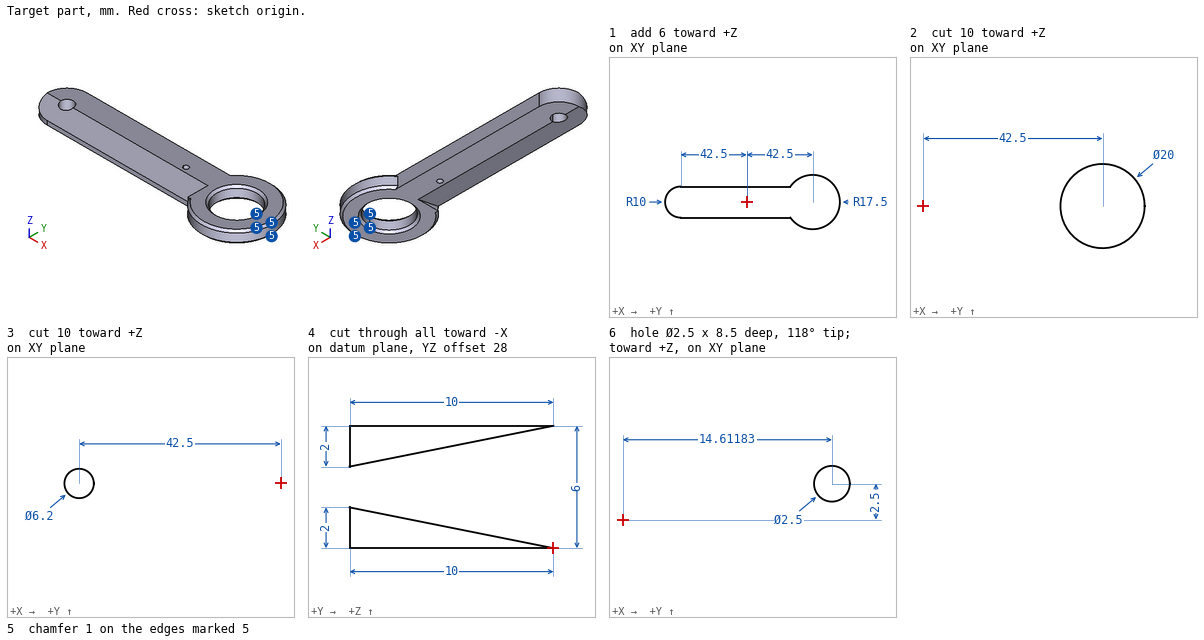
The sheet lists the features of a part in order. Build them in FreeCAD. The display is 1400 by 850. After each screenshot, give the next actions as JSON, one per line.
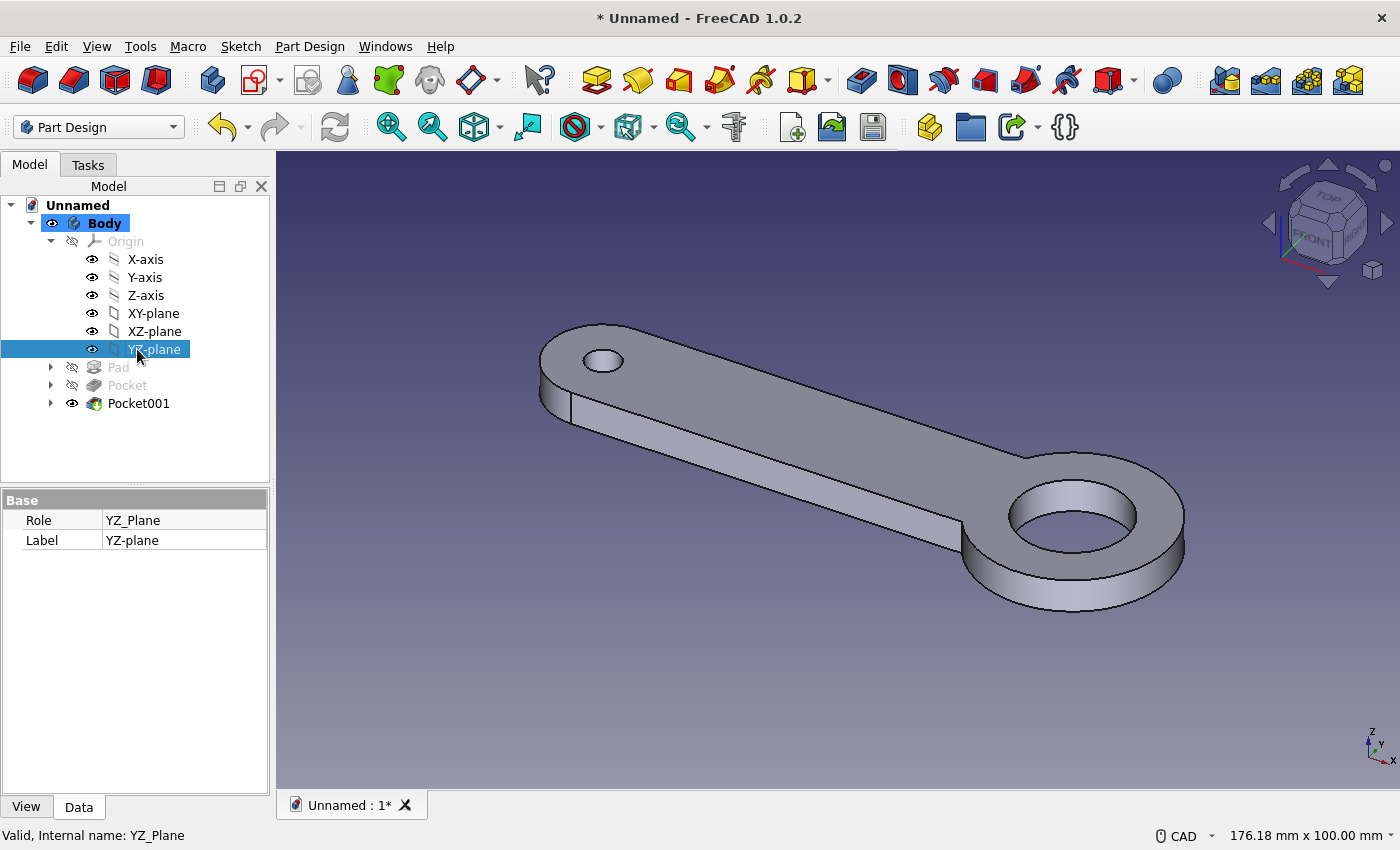
{"action": "left_click", "coordinate": [470, 80]}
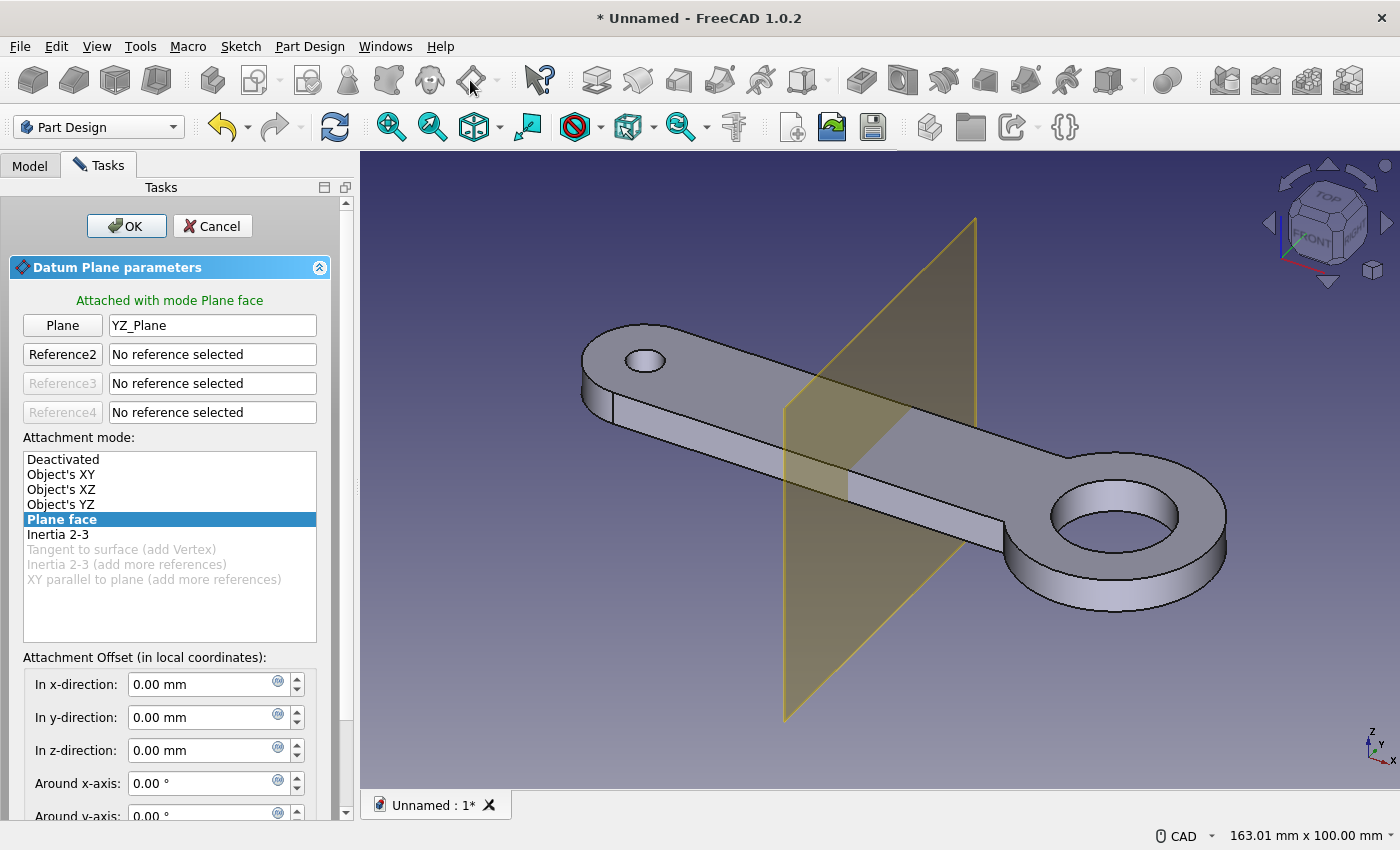
{"action": "triple_click", "coordinate": [210, 750]}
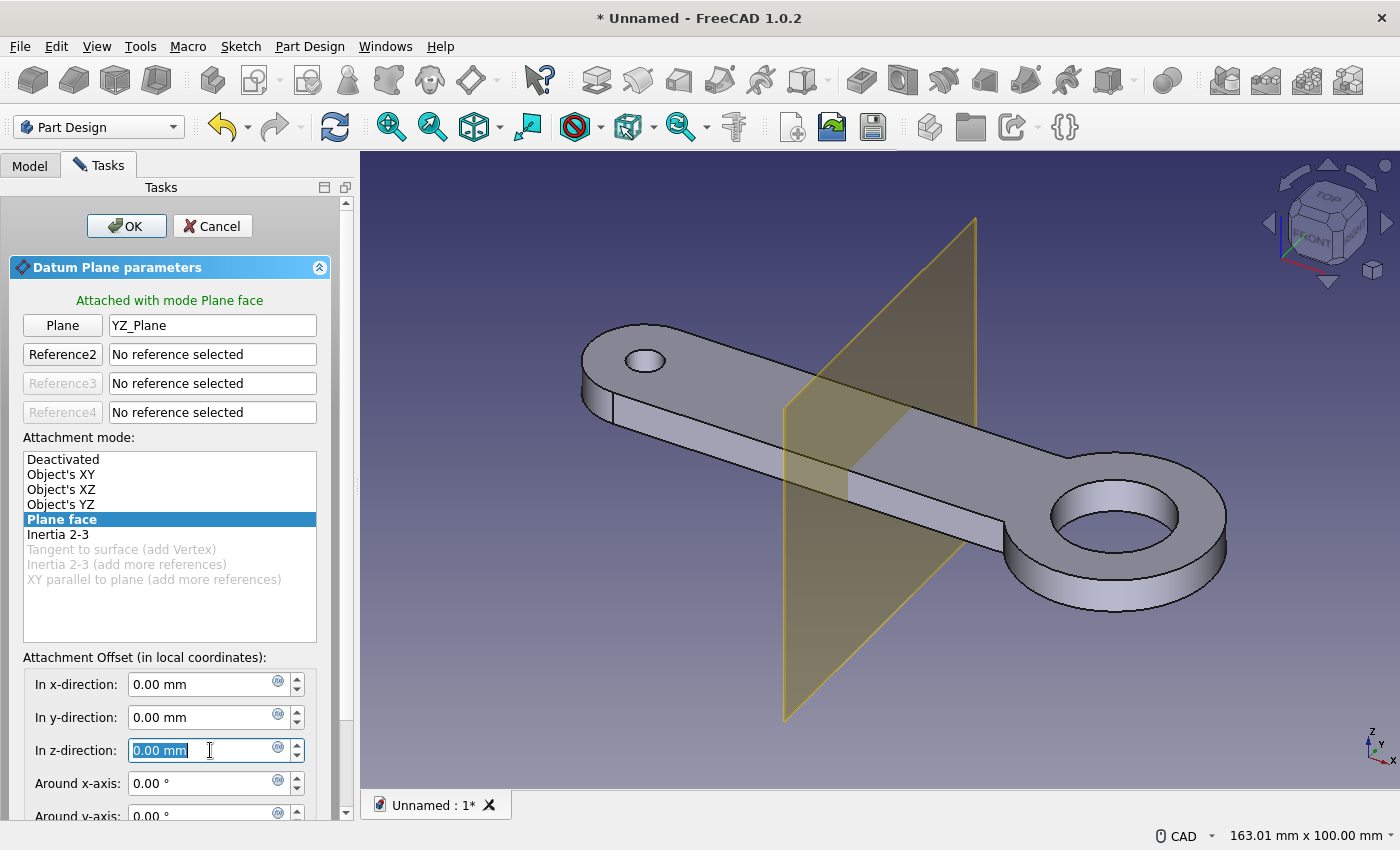
{"action": "type", "text": "28"}
{"action": "key", "text": "Tab"}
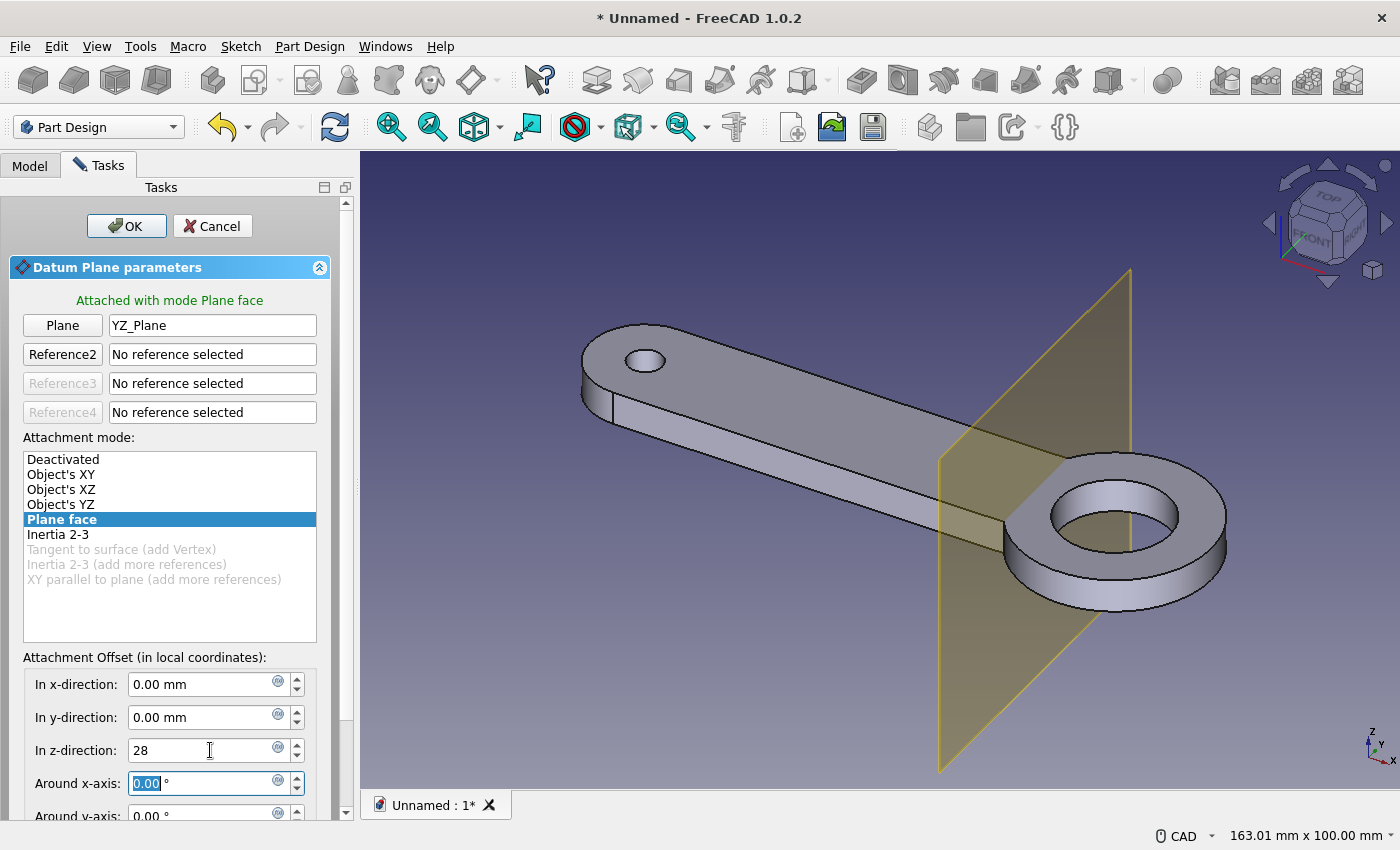
{"action": "left_click", "coordinate": [127, 226]}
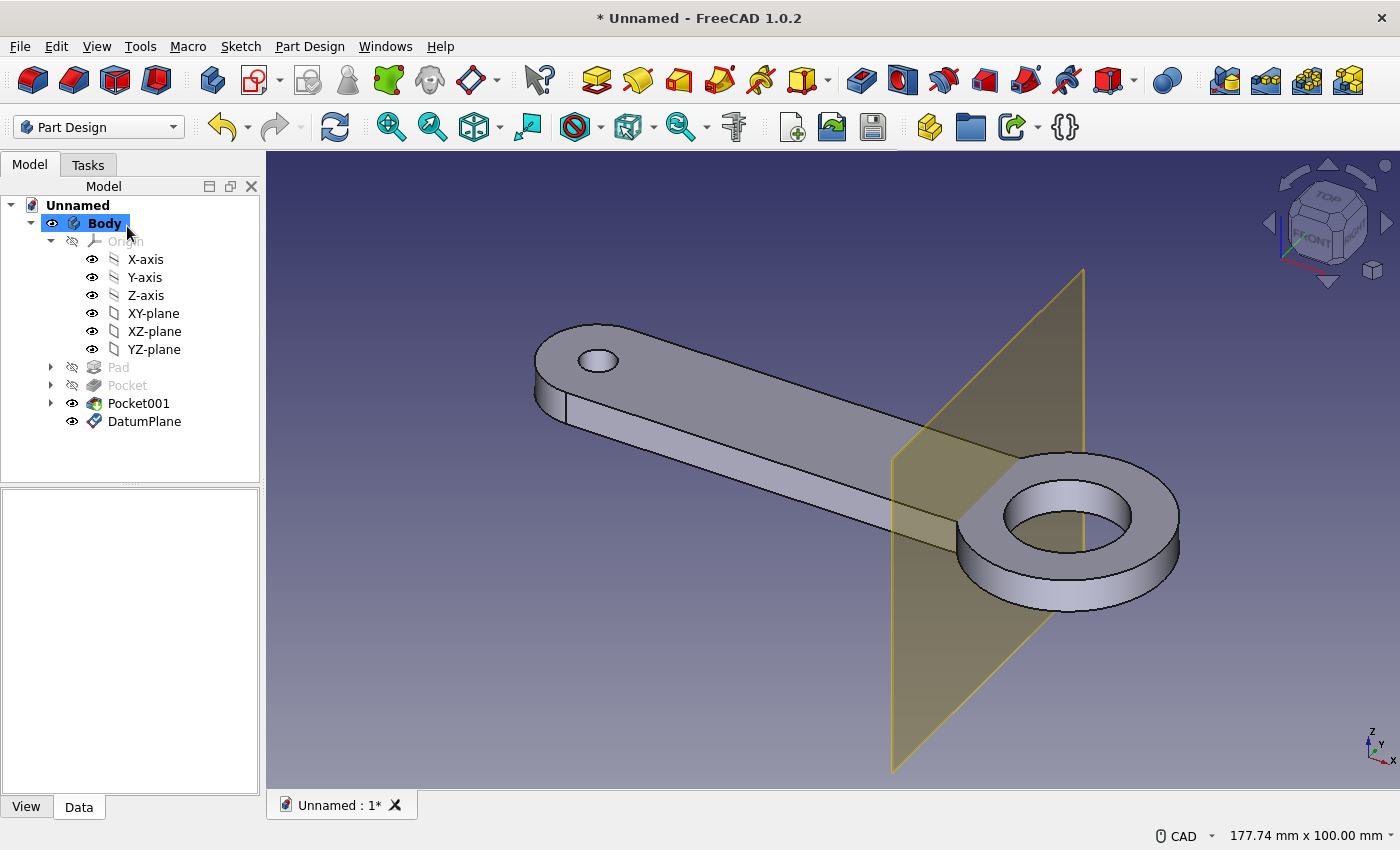
{"action": "left_click", "coordinate": [117, 421]}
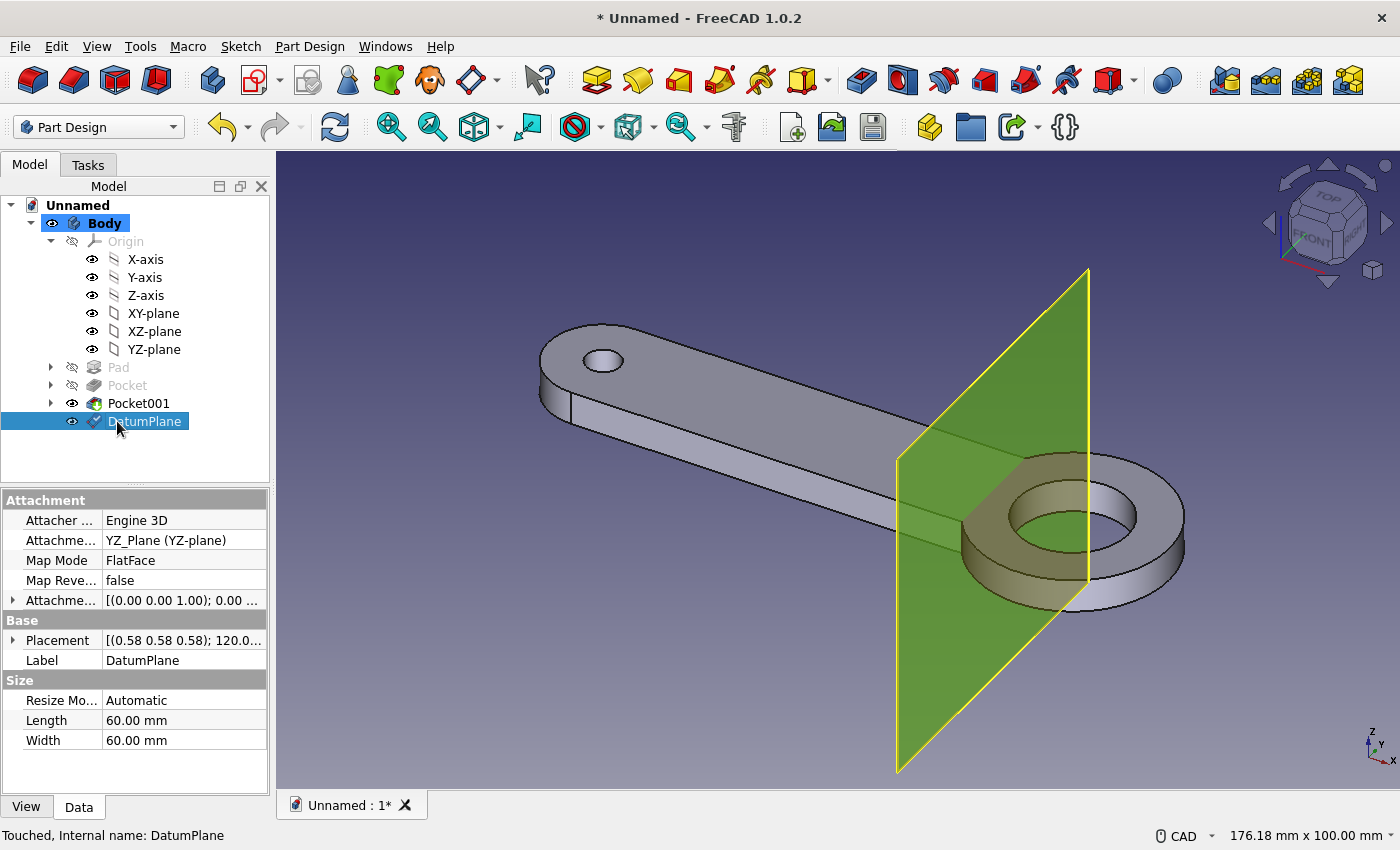
{"action": "left_click", "coordinate": [254, 80]}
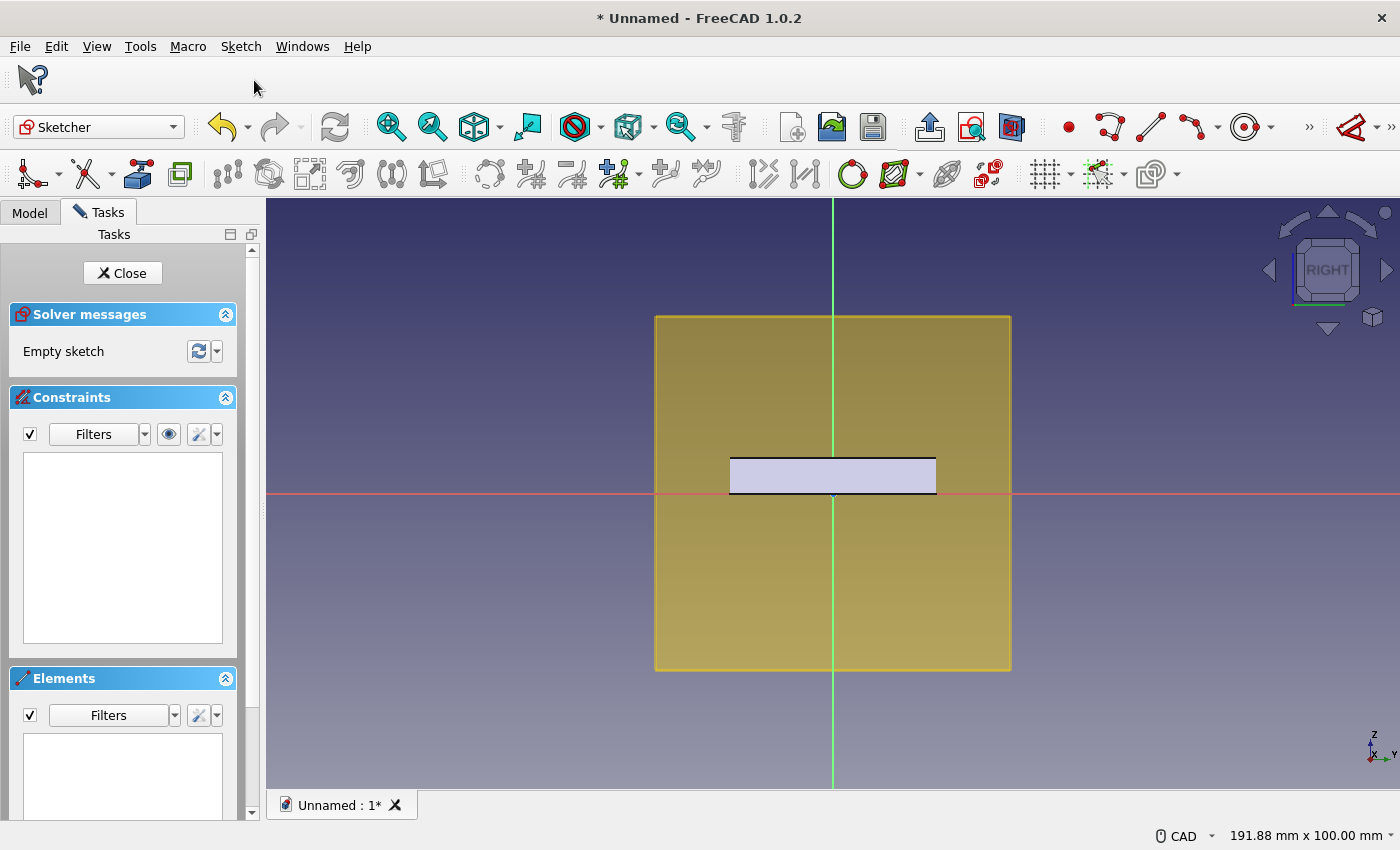
{"action": "key", "text": "q s"}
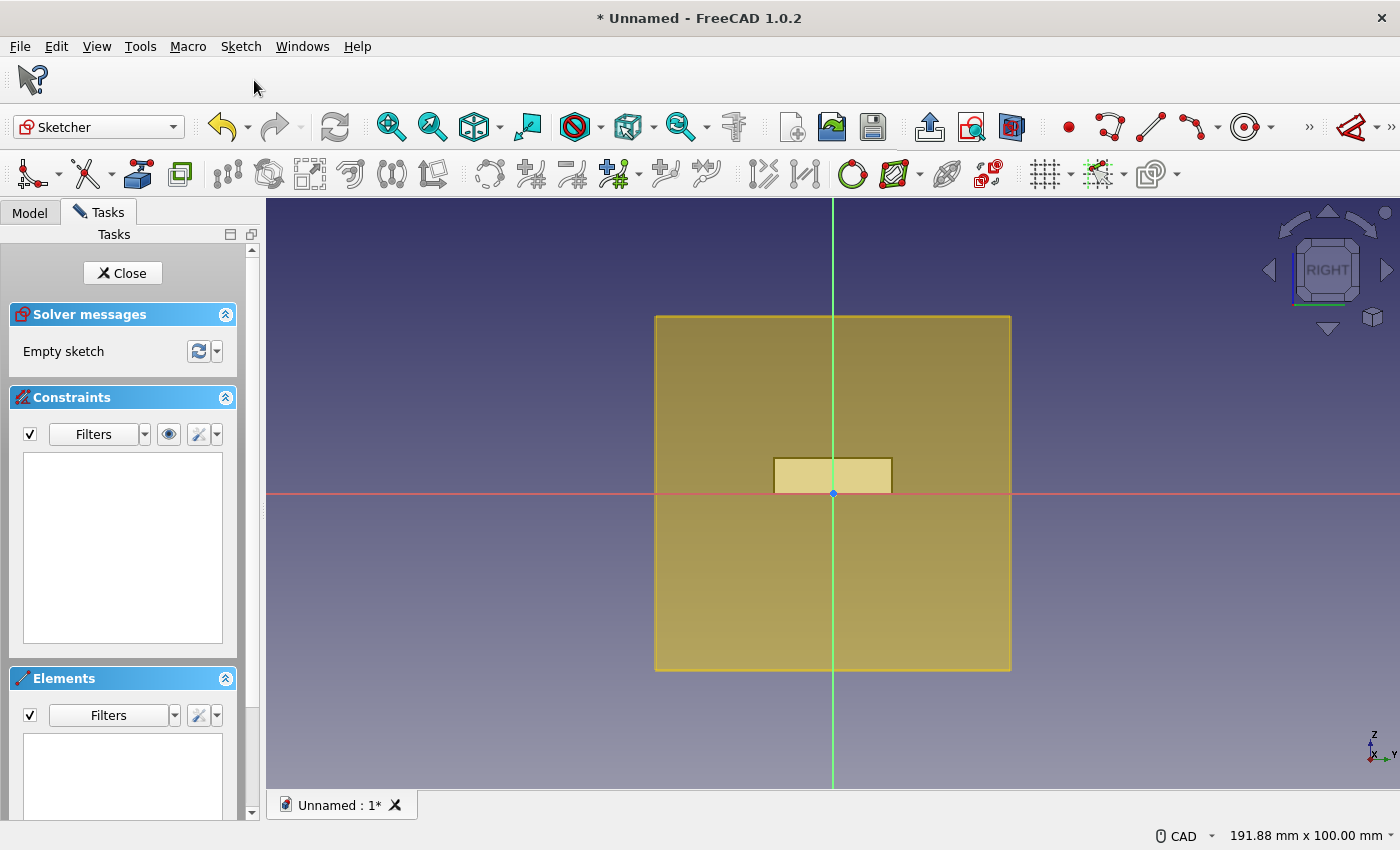
{"action": "scroll", "coordinate": [807, 474], "scroll_direction": "up", "scroll_amount": 12}